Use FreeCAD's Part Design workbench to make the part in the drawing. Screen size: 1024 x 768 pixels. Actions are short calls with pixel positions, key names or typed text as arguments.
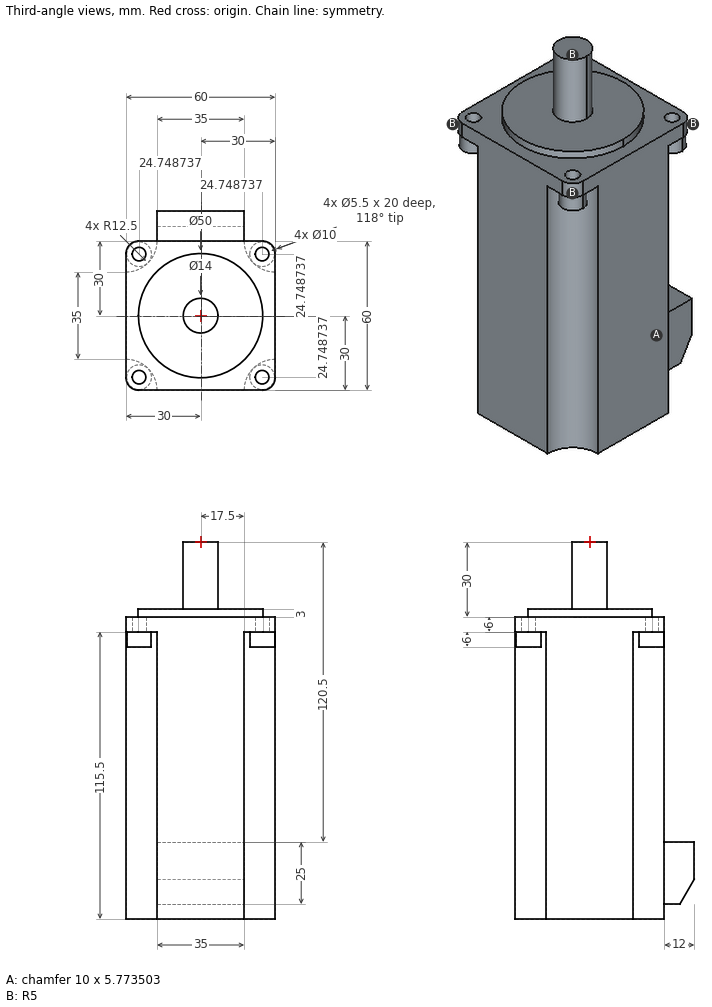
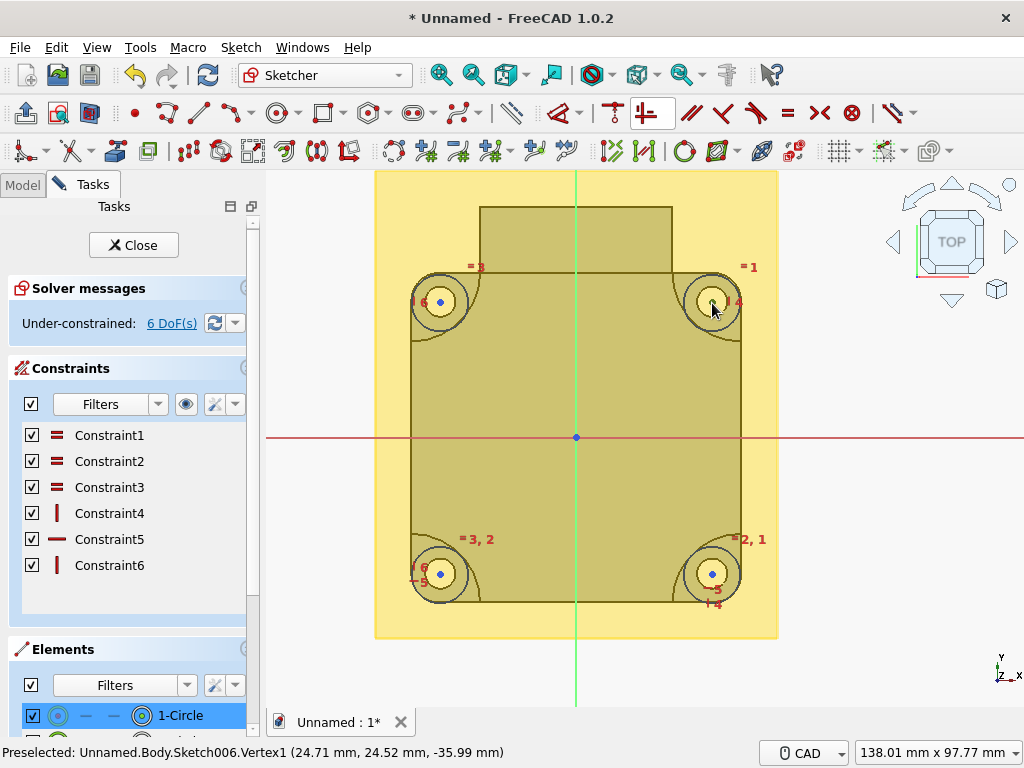
click(440, 303)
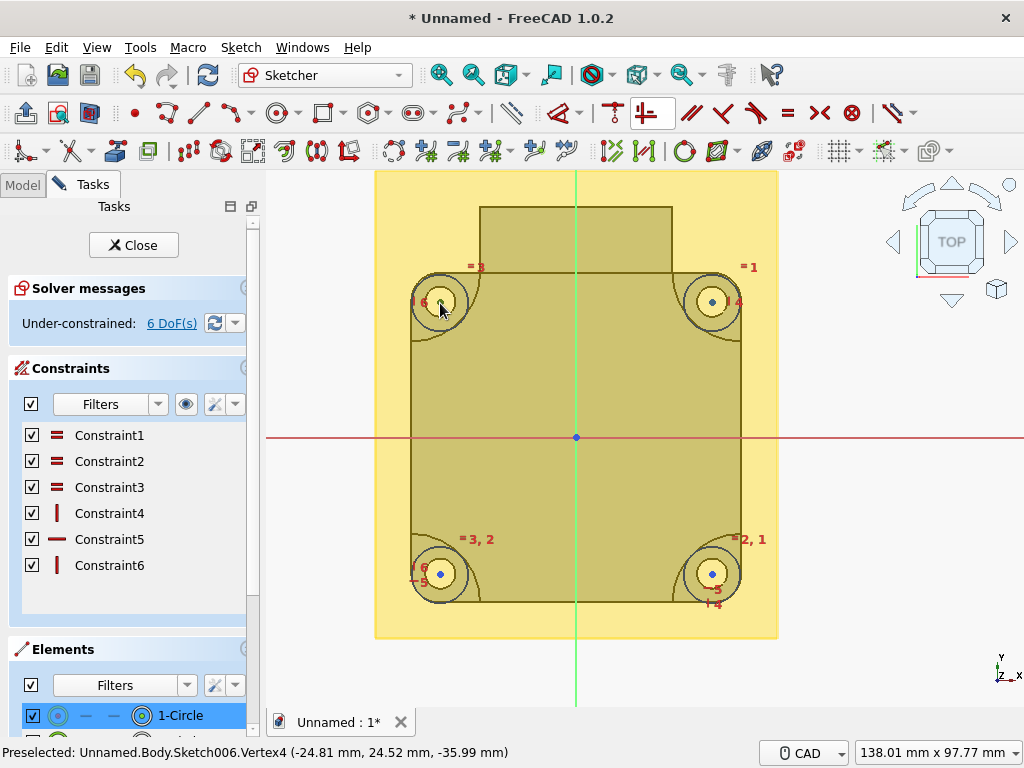
click(670, 114)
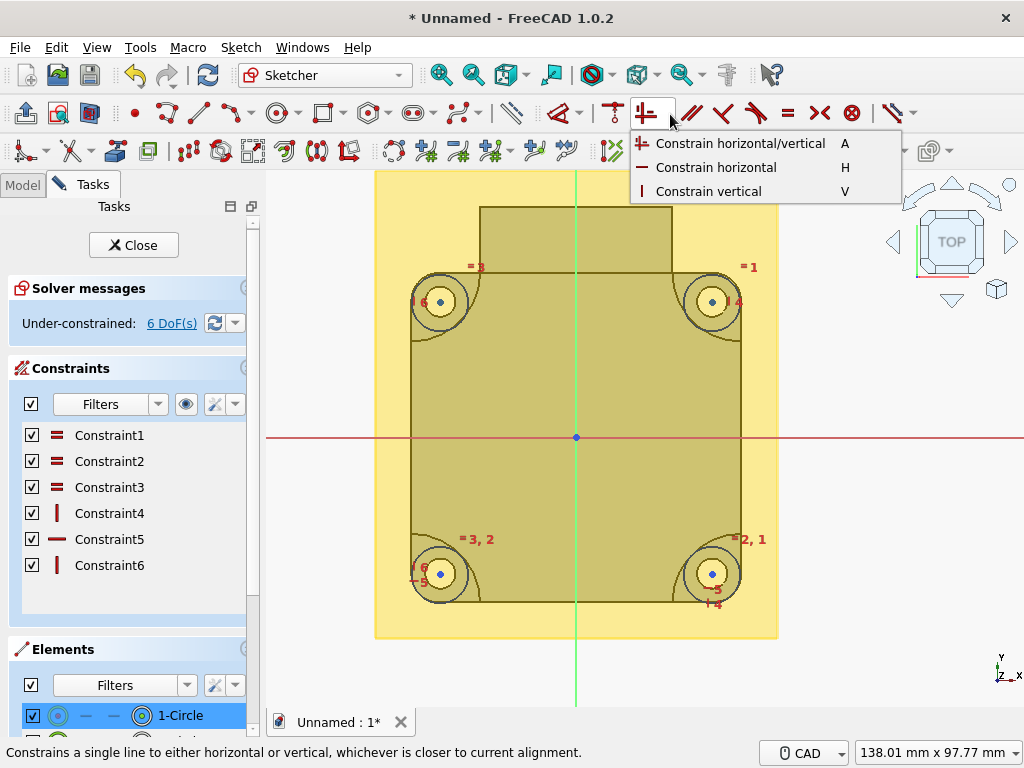
click(766, 167)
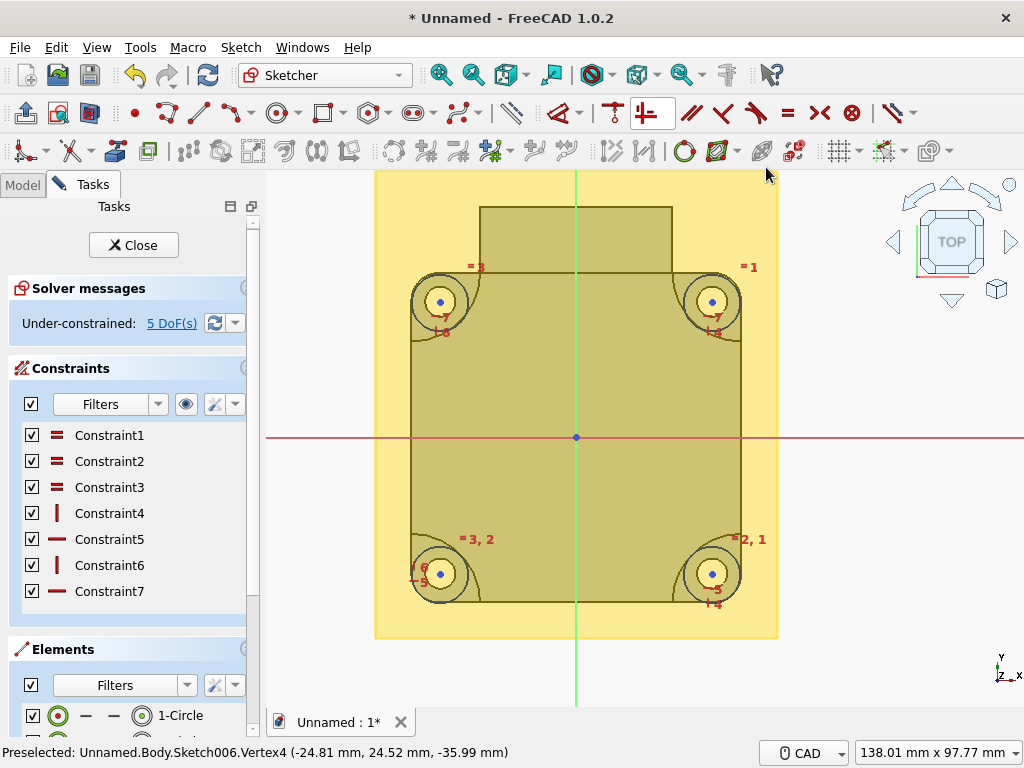
click(558, 114)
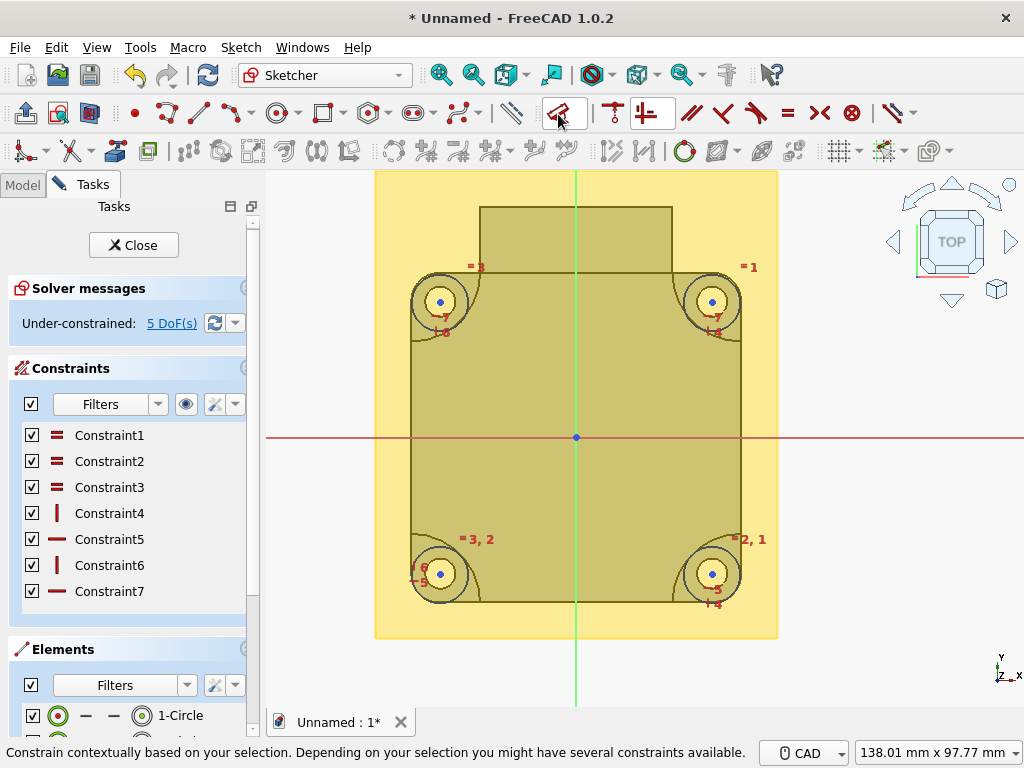
click(732, 283)
click(755, 260)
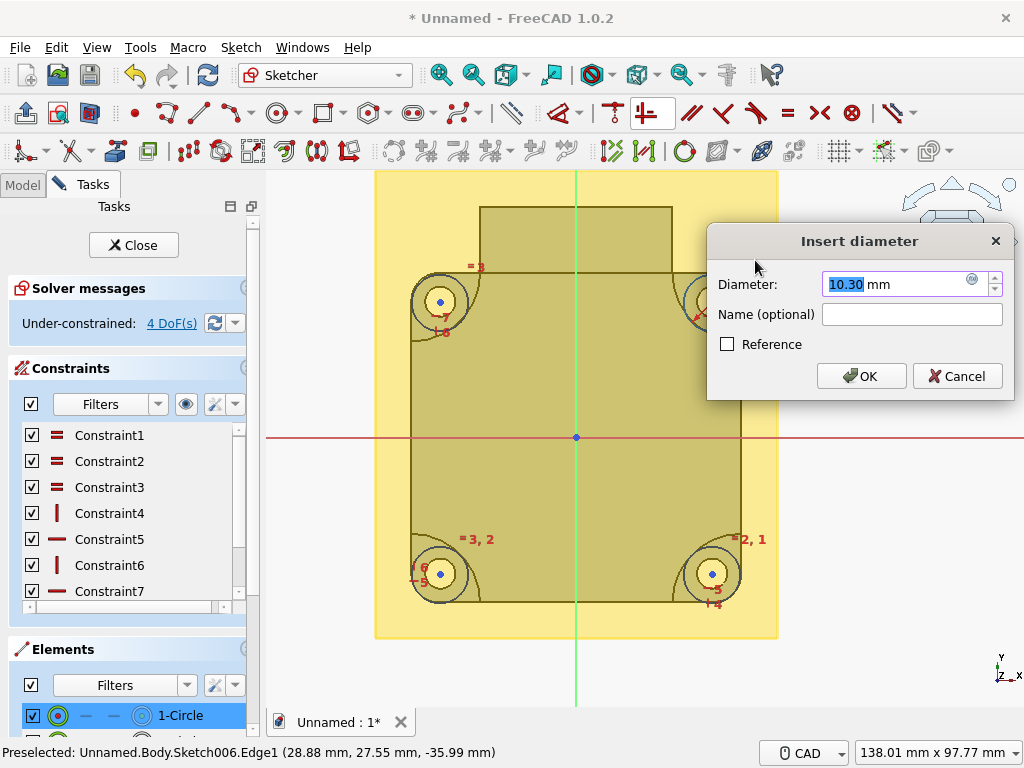
text(10)
key(Return)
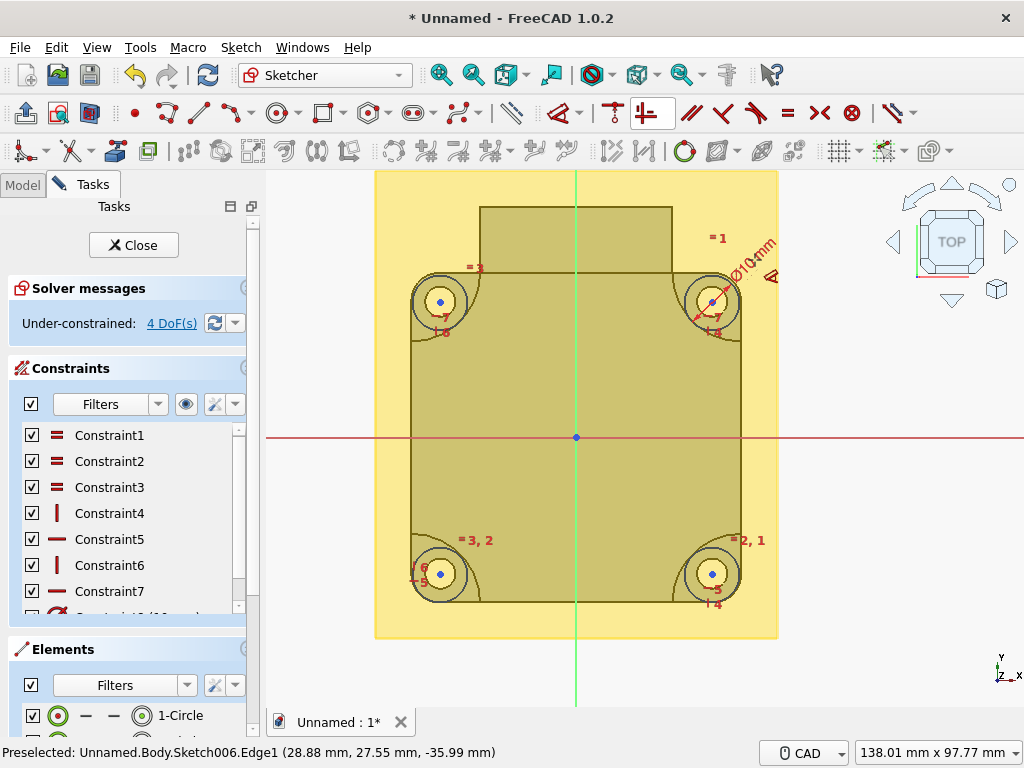
click(712, 303)
click(644, 269)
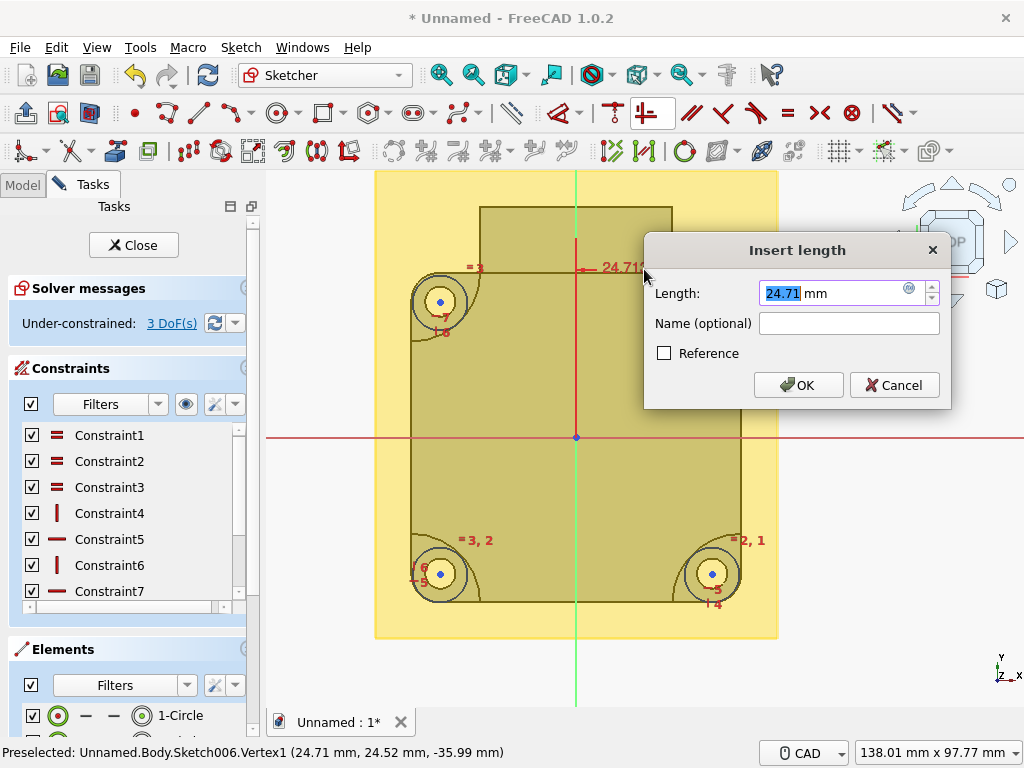
text(24.748737)
key(Return)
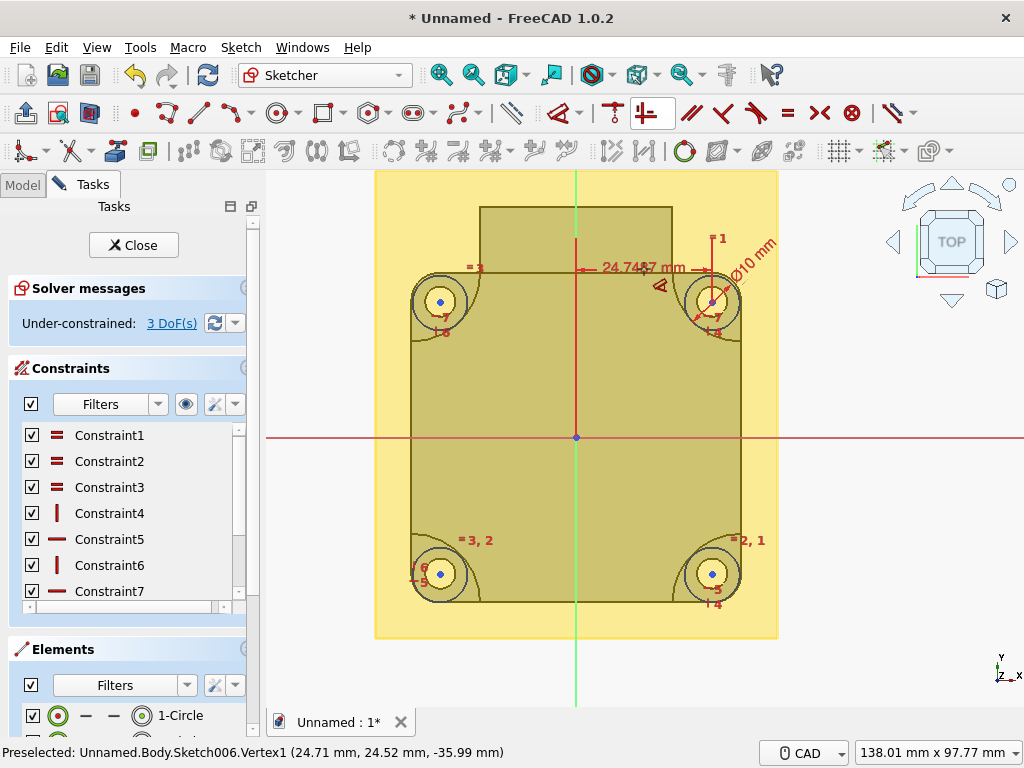
click(712, 303)
click(746, 370)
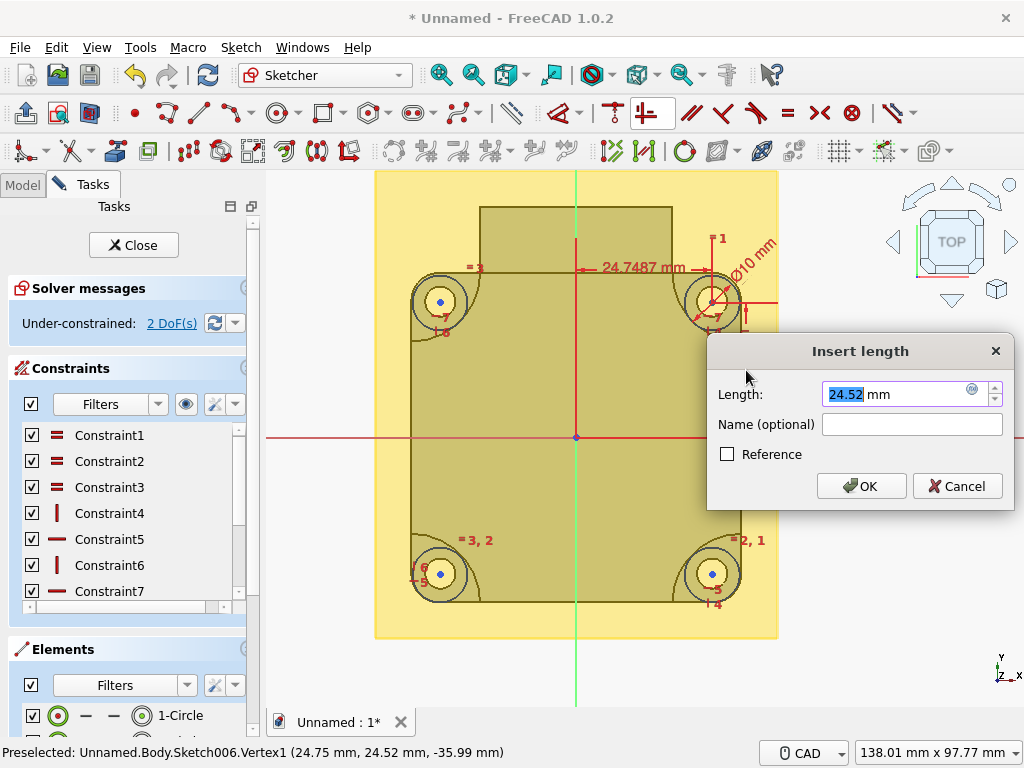
text(24.748737)
key(Return)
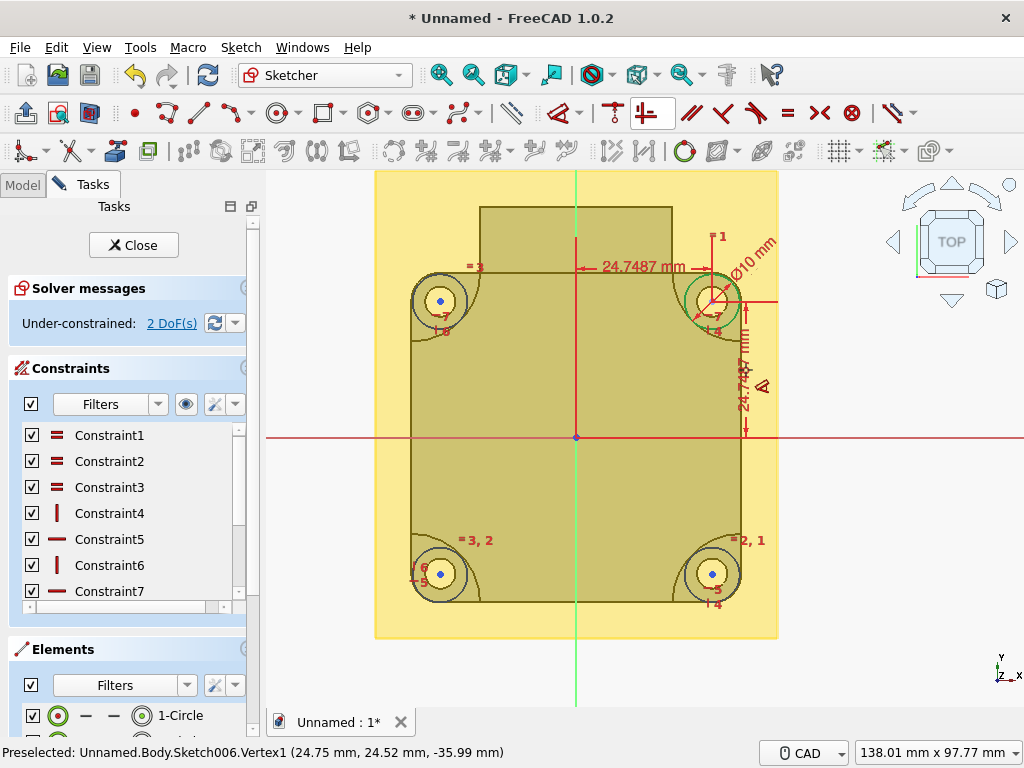
click(712, 575)
click(746, 506)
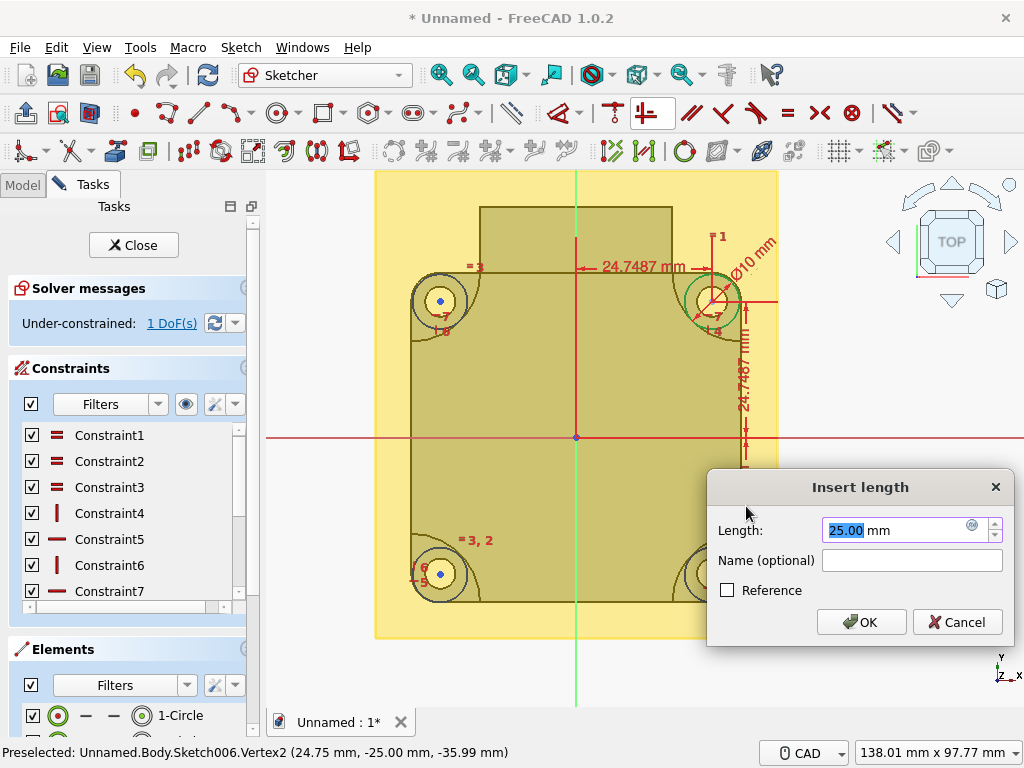
text(24.748737)
key(Return)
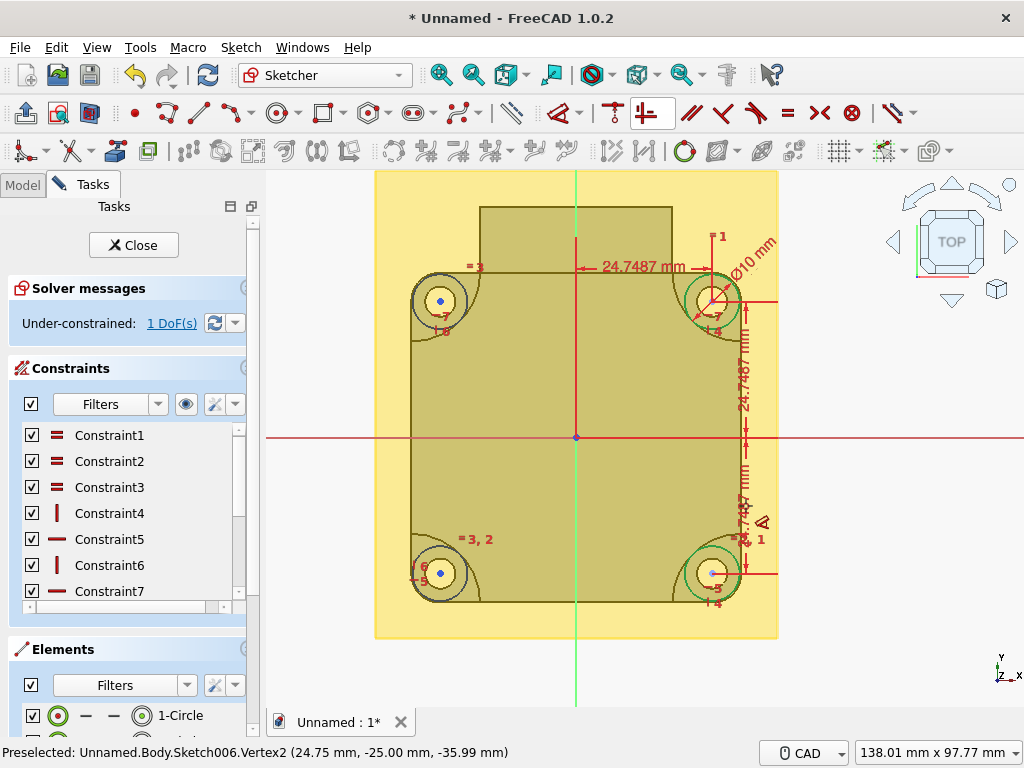
click(440, 574)
click(508, 608)